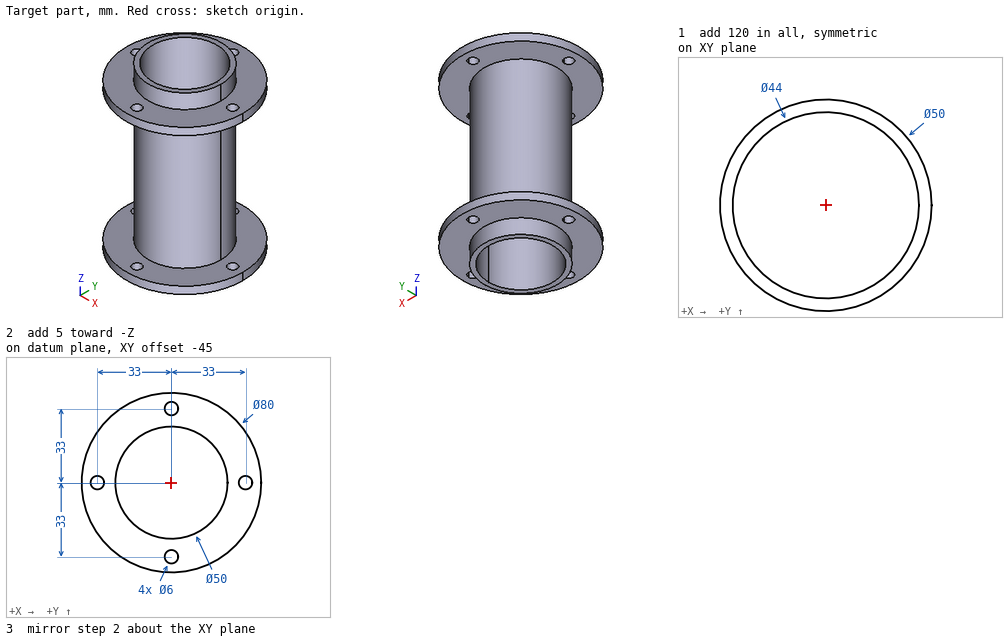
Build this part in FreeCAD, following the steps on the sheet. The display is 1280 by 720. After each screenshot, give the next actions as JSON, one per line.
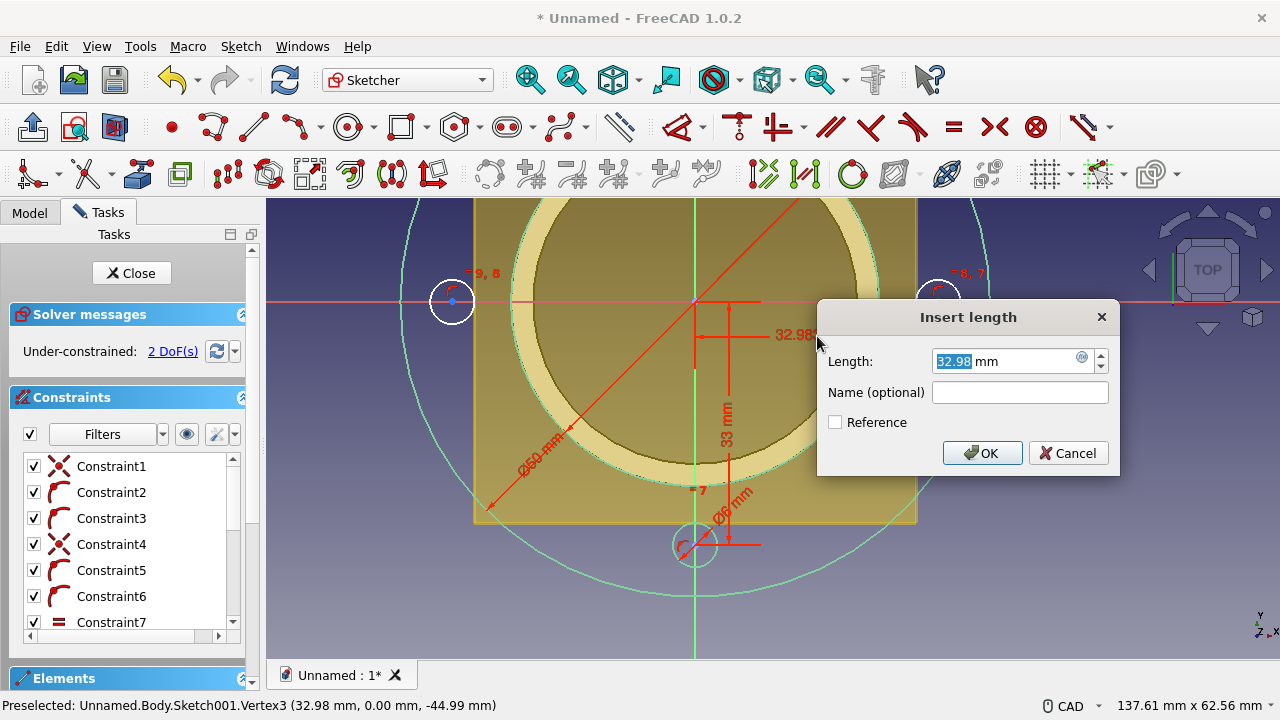
{"action": "type", "text": "33"}
{"action": "key", "text": "Return"}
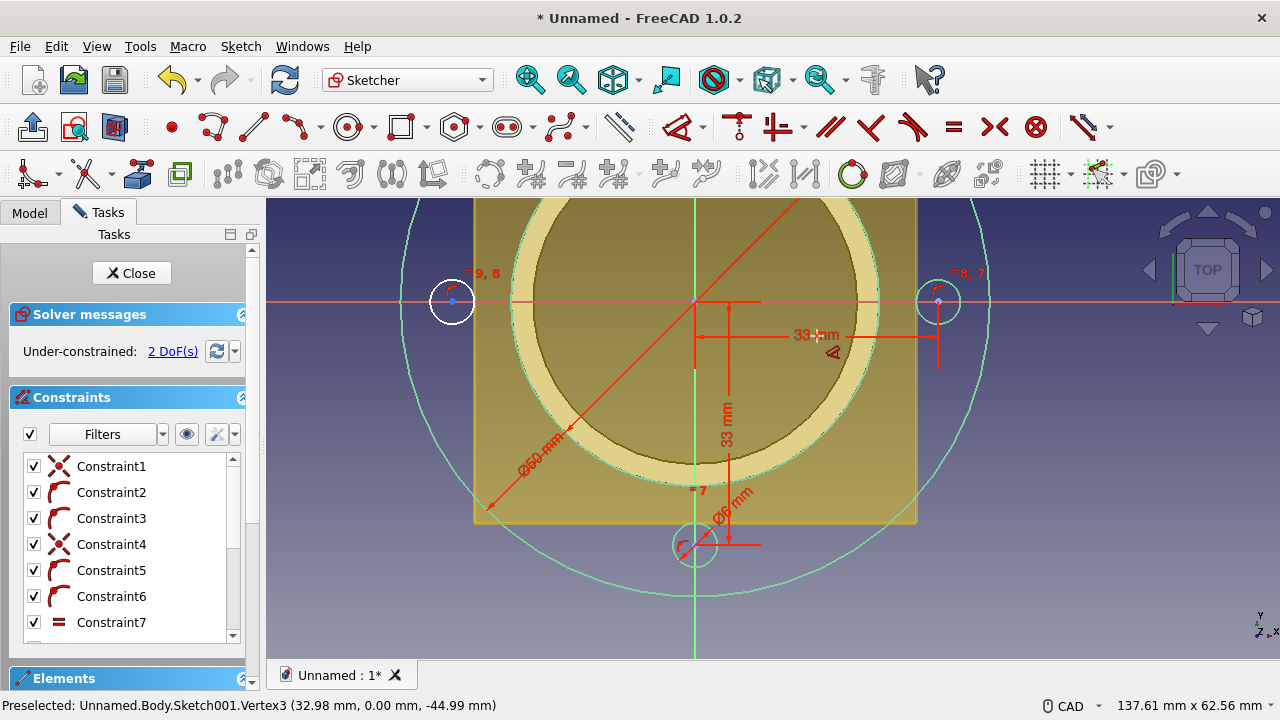
{"action": "left_click", "coordinate": [452, 302]}
{"action": "left_click", "coordinate": [574, 336]}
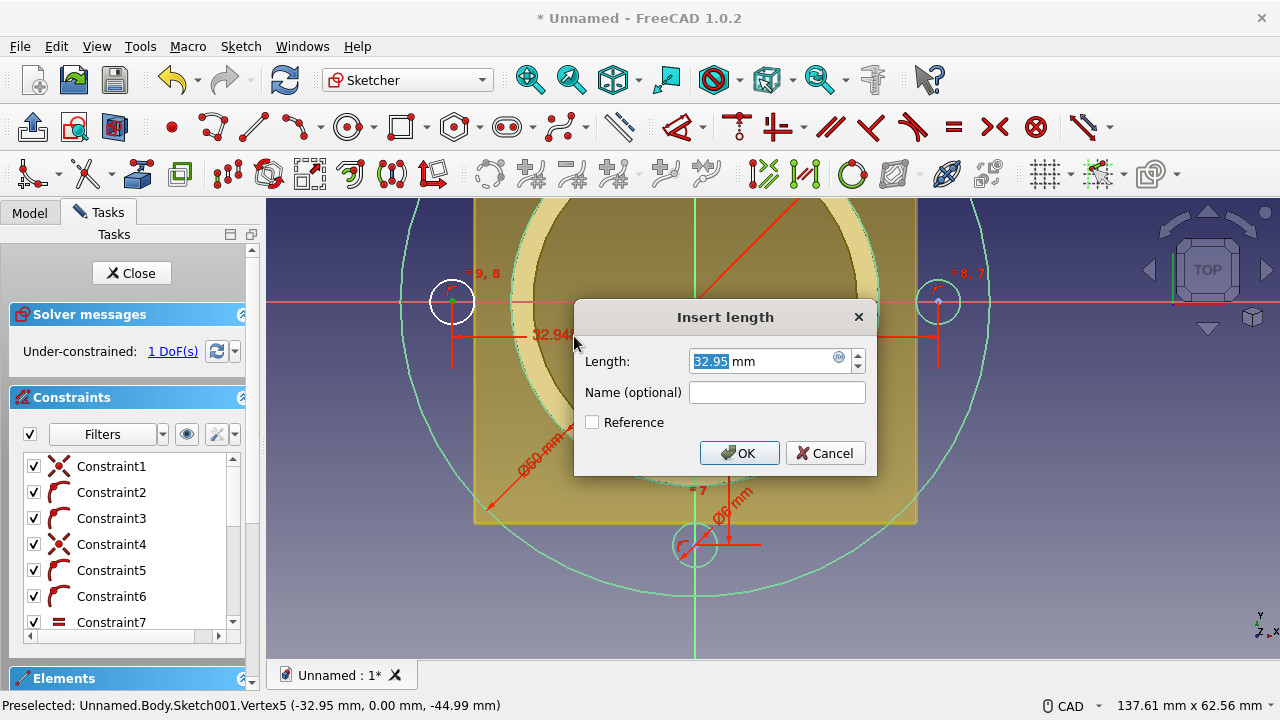
{"action": "type", "text": "33"}
{"action": "key", "text": "Return"}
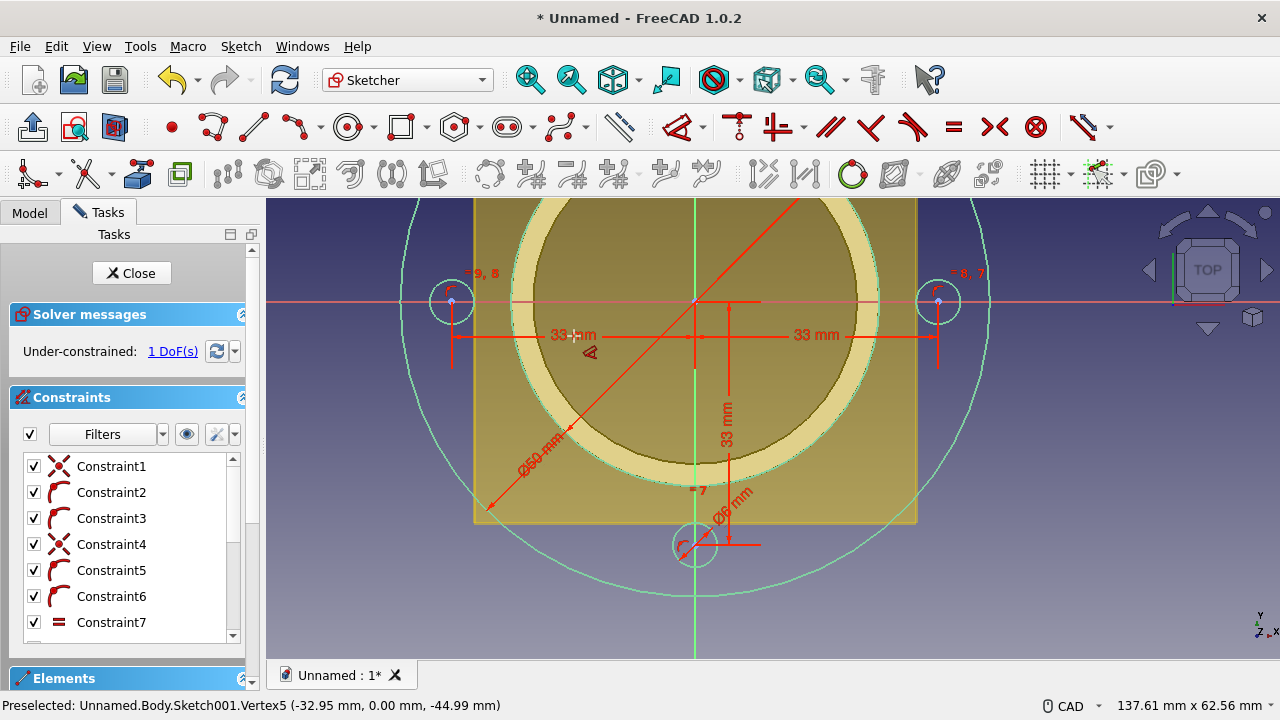
{"action": "scroll", "coordinate": [712, 532], "scroll_direction": "down", "scroll_amount": 4}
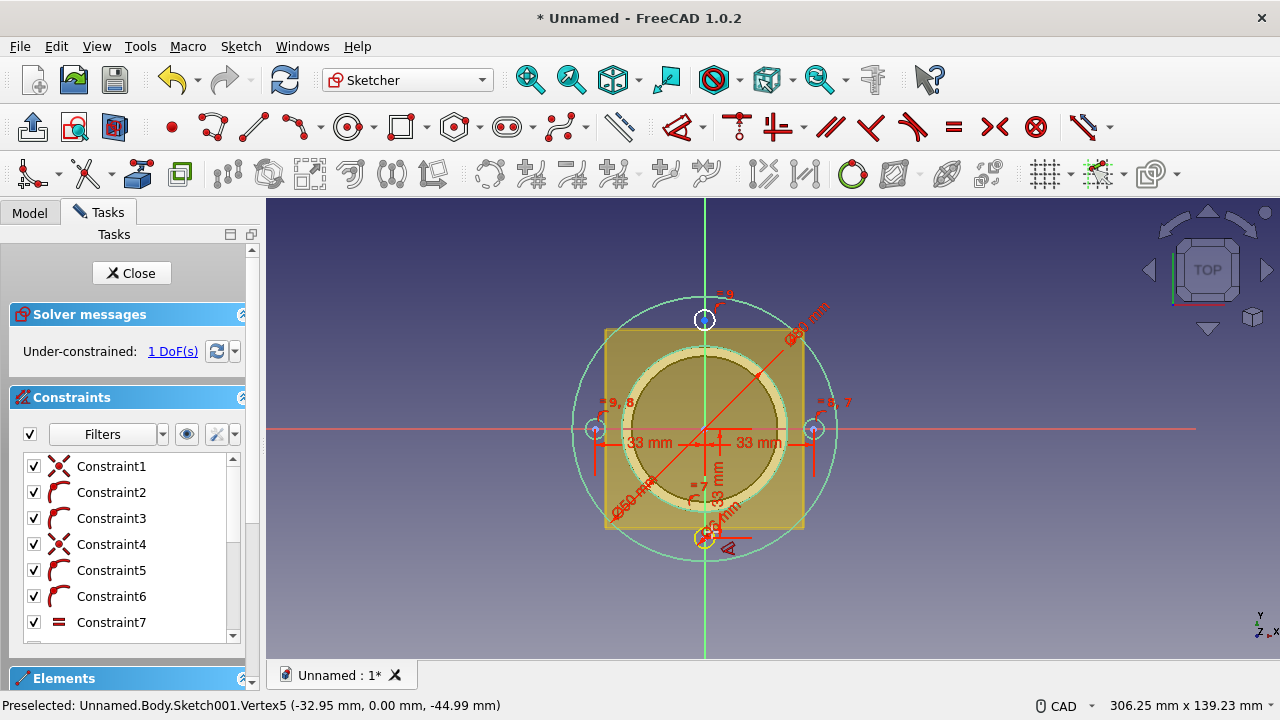
{"action": "left_click", "coordinate": [705, 320]}
{"action": "left_click", "coordinate": [739, 375]}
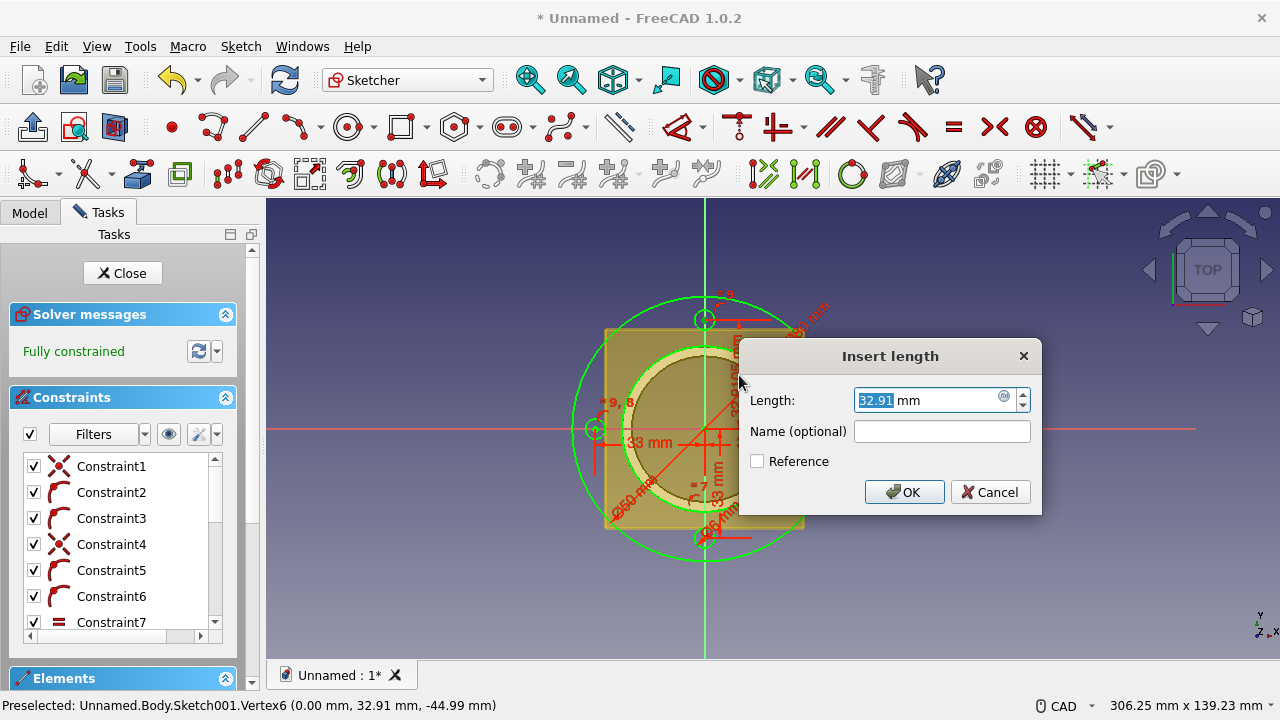
{"action": "type", "text": "33"}
{"action": "key", "text": "Return"}
{"action": "key", "text": "Escape"}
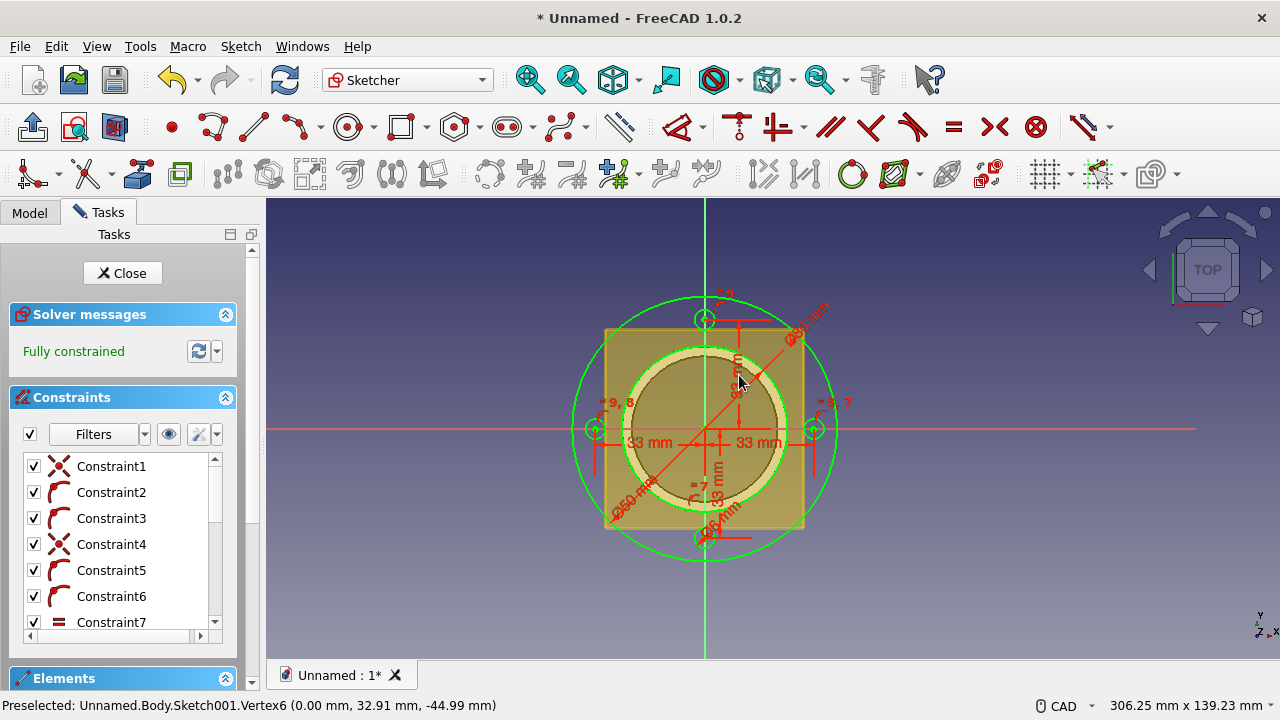
{"action": "left_click", "coordinate": [123, 273]}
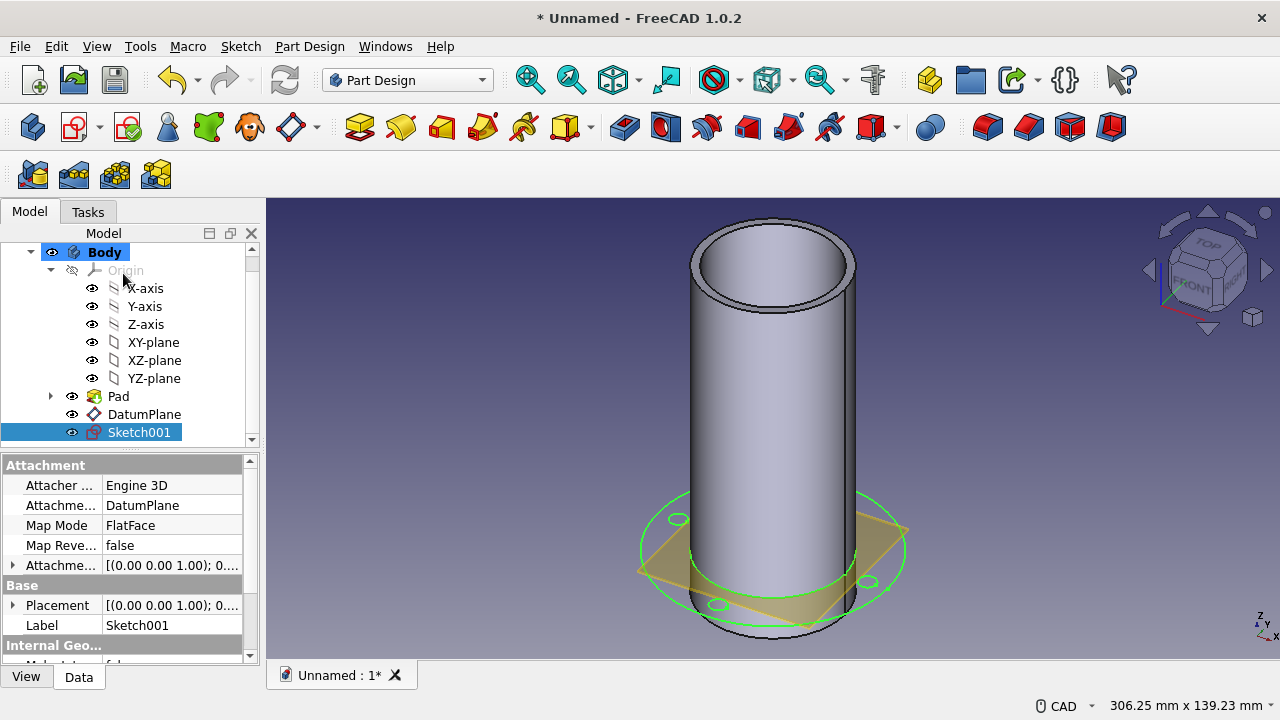
{"action": "left_click", "coordinate": [360, 128]}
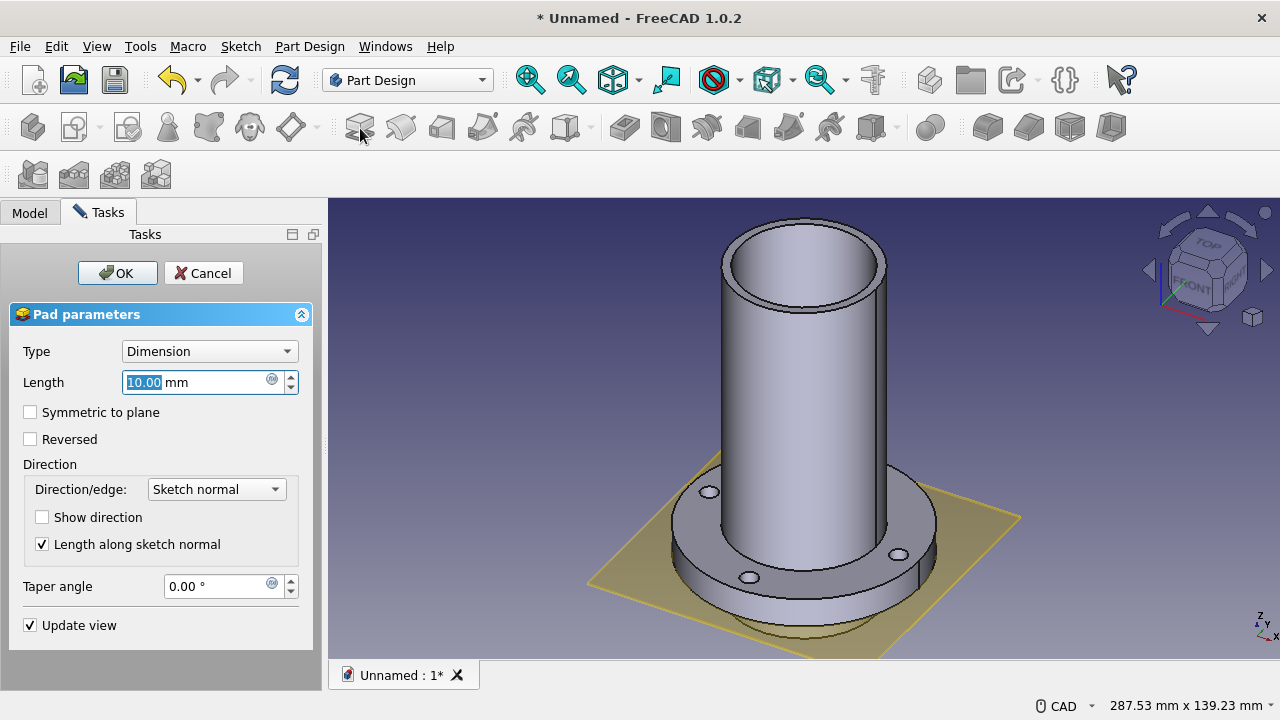
{"action": "type", "text": "5"}
{"action": "key", "text": "Tab"}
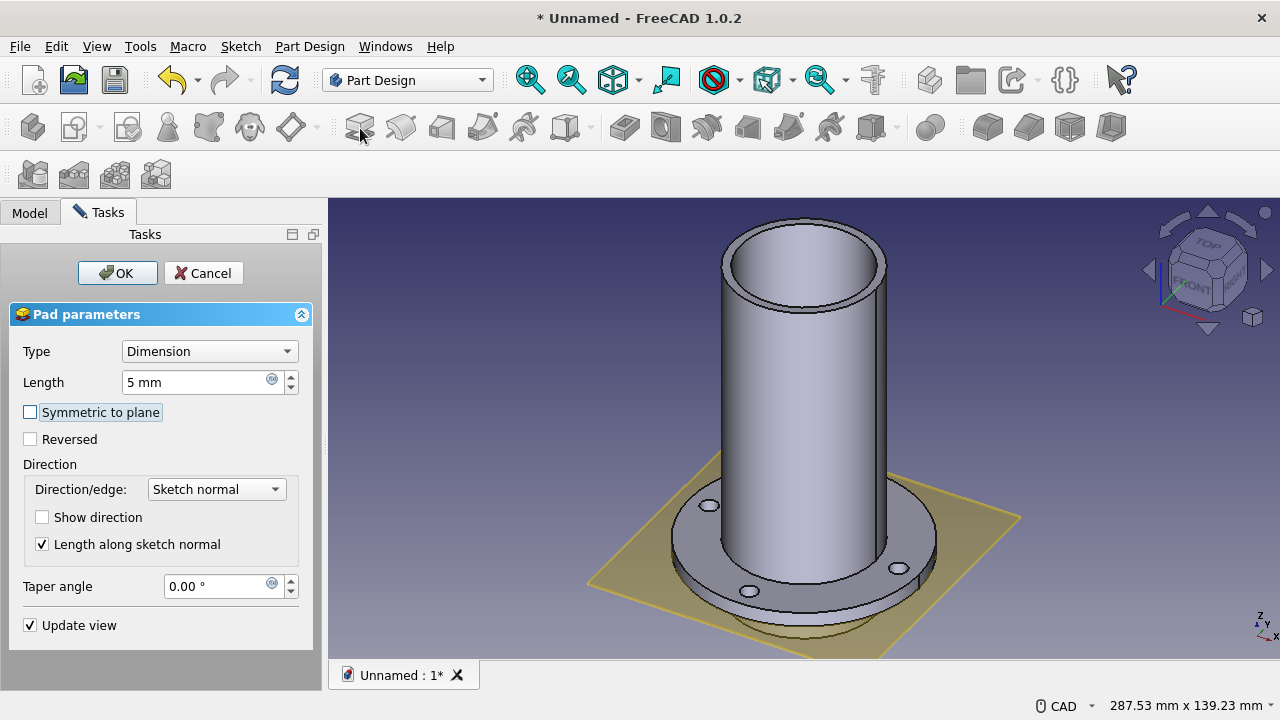
{"action": "left_click", "coordinate": [31, 439]}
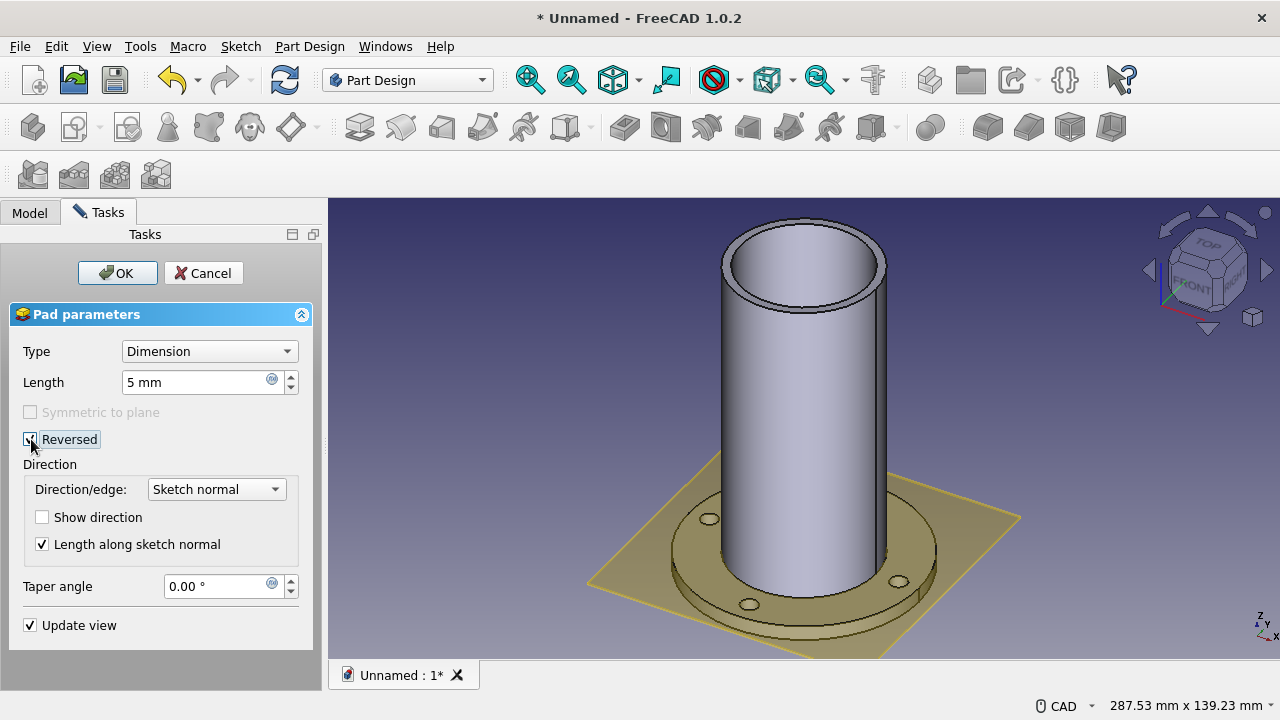
{"action": "left_click", "coordinate": [118, 273]}